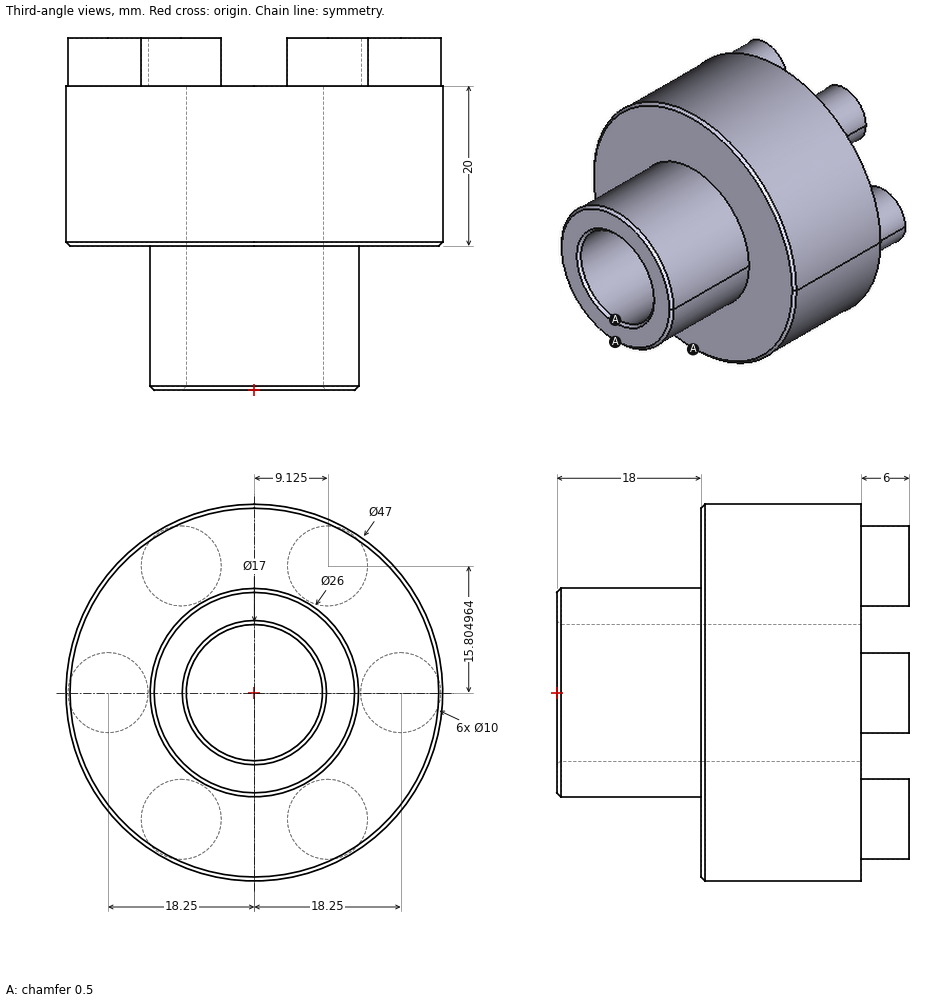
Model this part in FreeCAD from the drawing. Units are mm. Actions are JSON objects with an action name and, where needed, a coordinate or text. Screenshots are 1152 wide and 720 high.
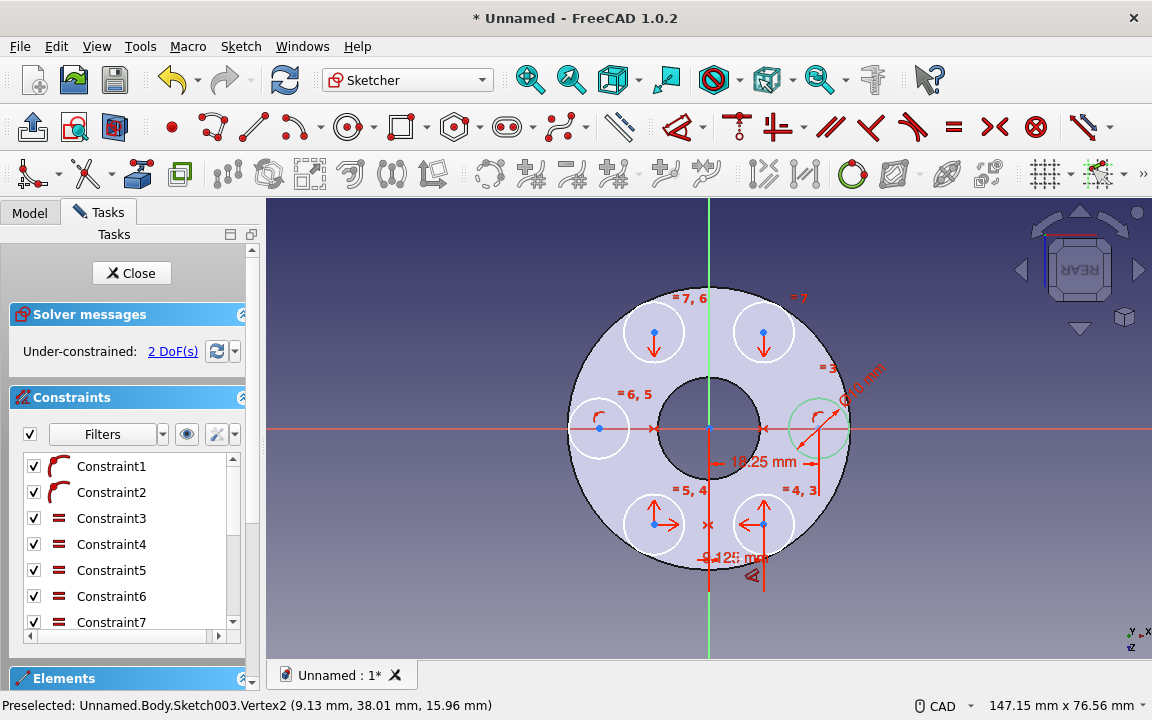
{"action": "left_click", "coordinate": [599, 429]}
{"action": "left_click", "coordinate": [654, 463]}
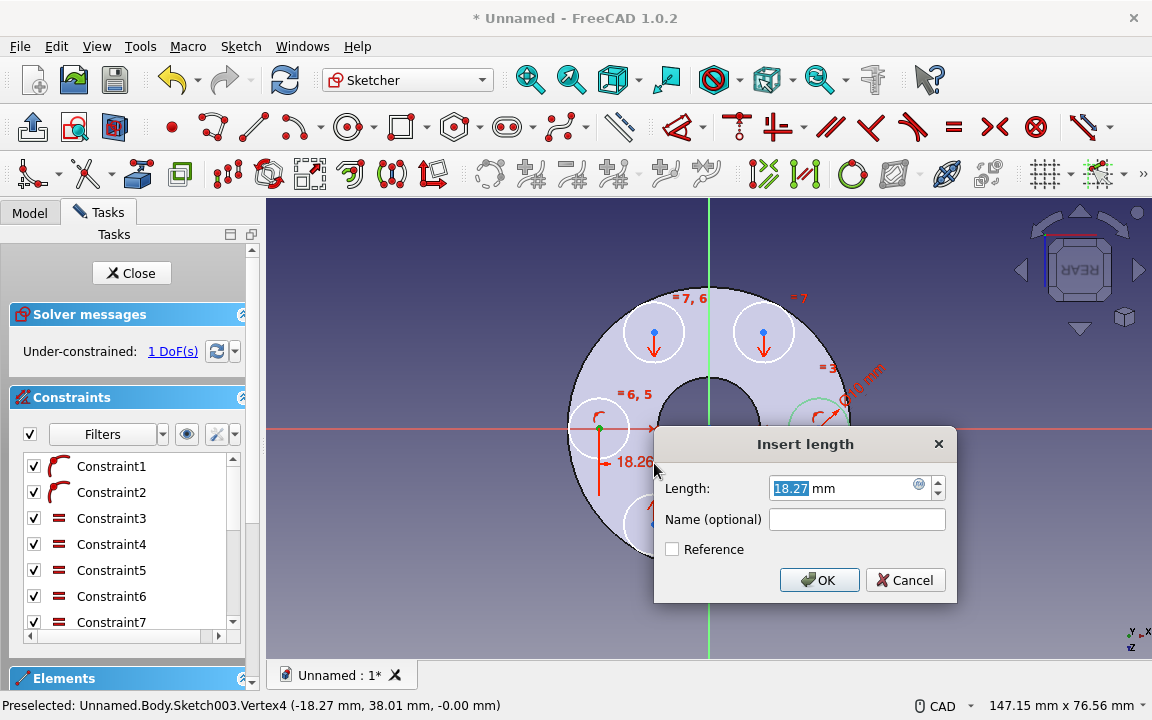
{"action": "type", "text": "18.25"}
{"action": "key", "text": "Return"}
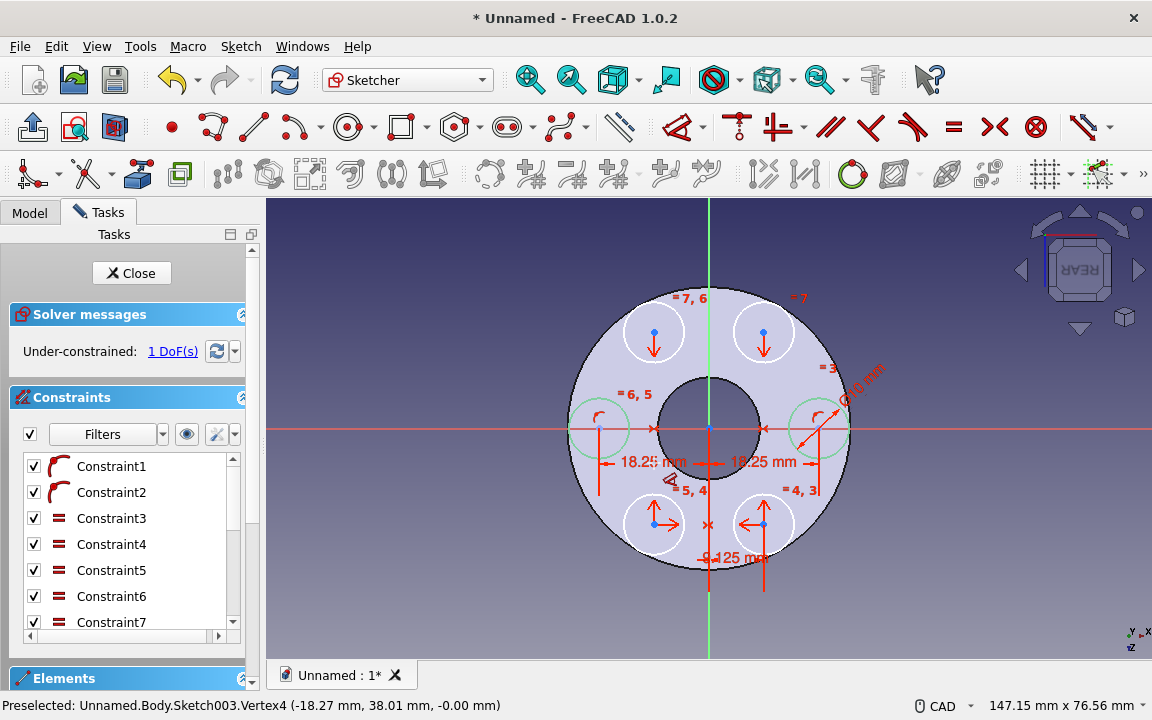
{"action": "left_click", "coordinate": [764, 525]}
{"action": "left_click", "coordinate": [822, 499]}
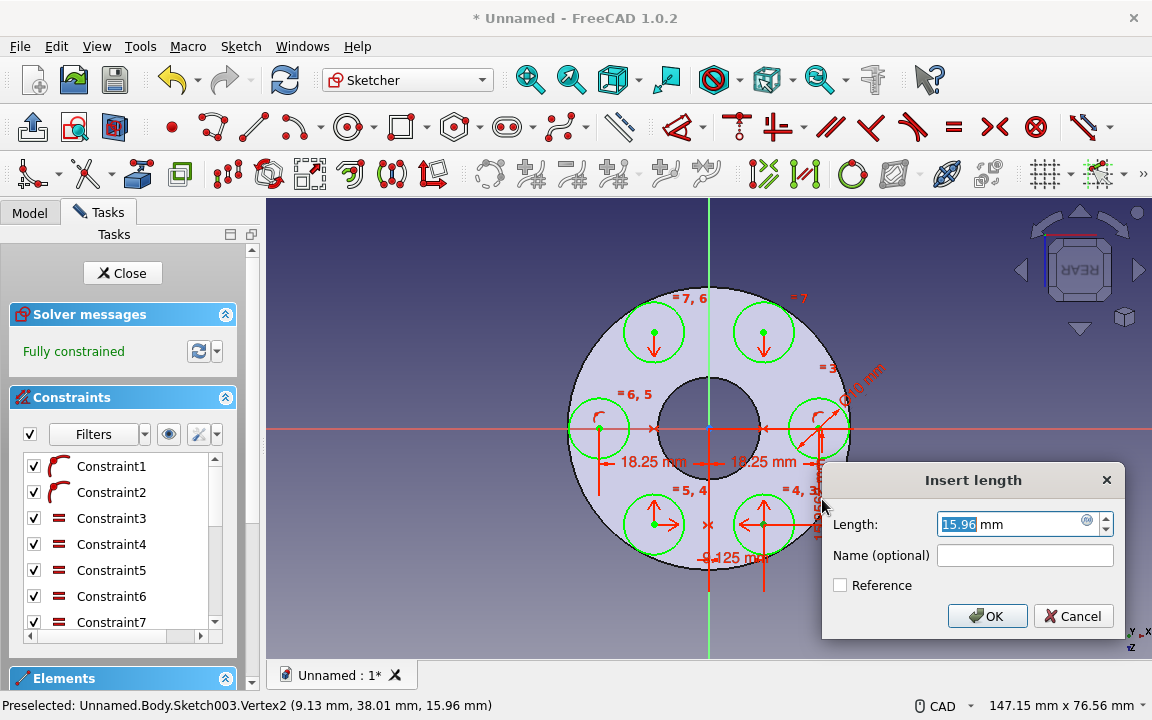
{"action": "type", "text": "15.804964"}
{"action": "key", "text": "Return"}
{"action": "key", "text": "Escape"}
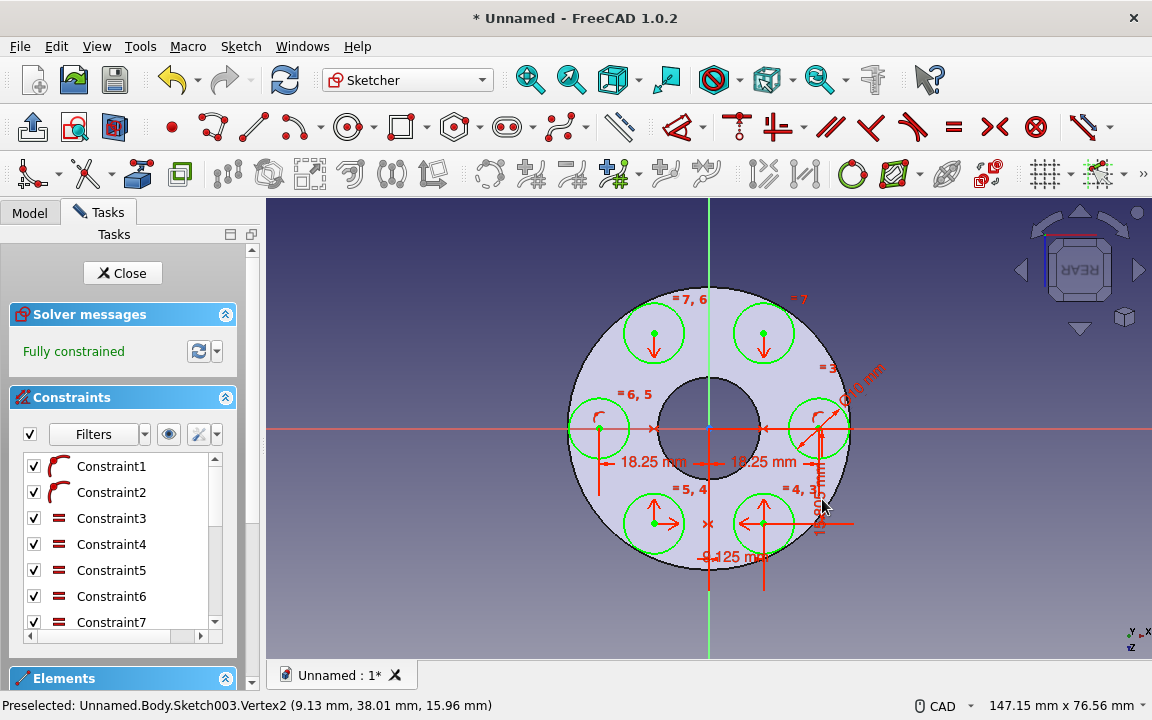
{"action": "left_click", "coordinate": [123, 273]}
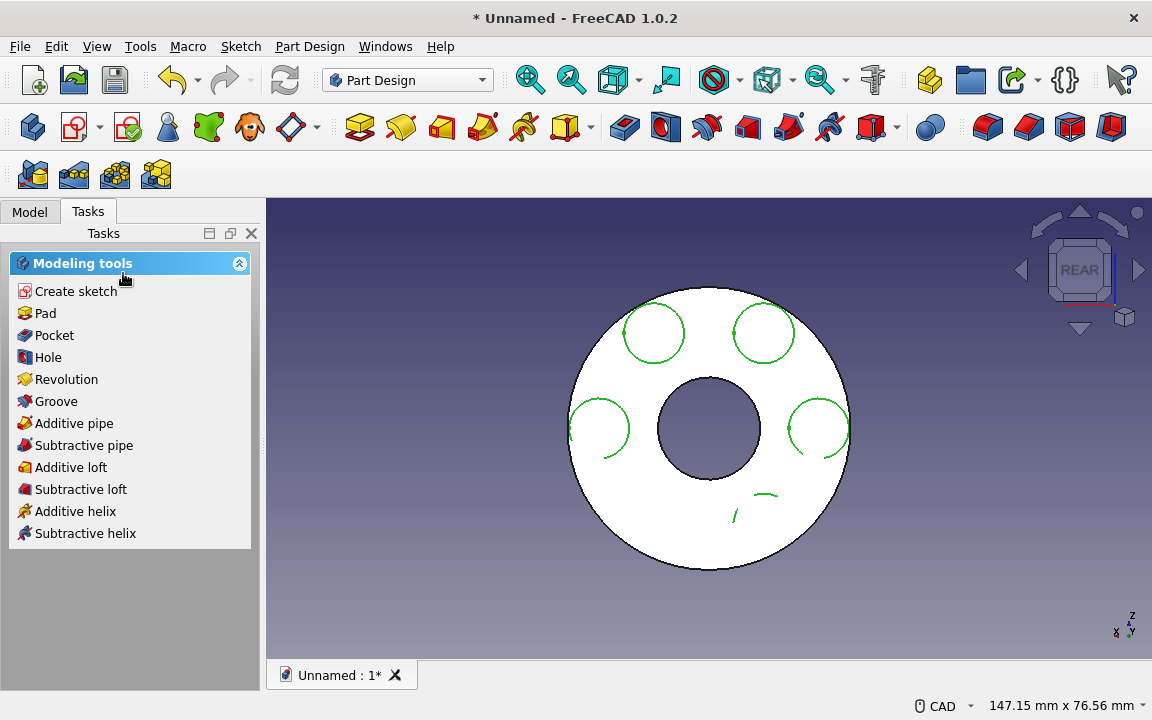
{"action": "left_click", "coordinate": [360, 128]}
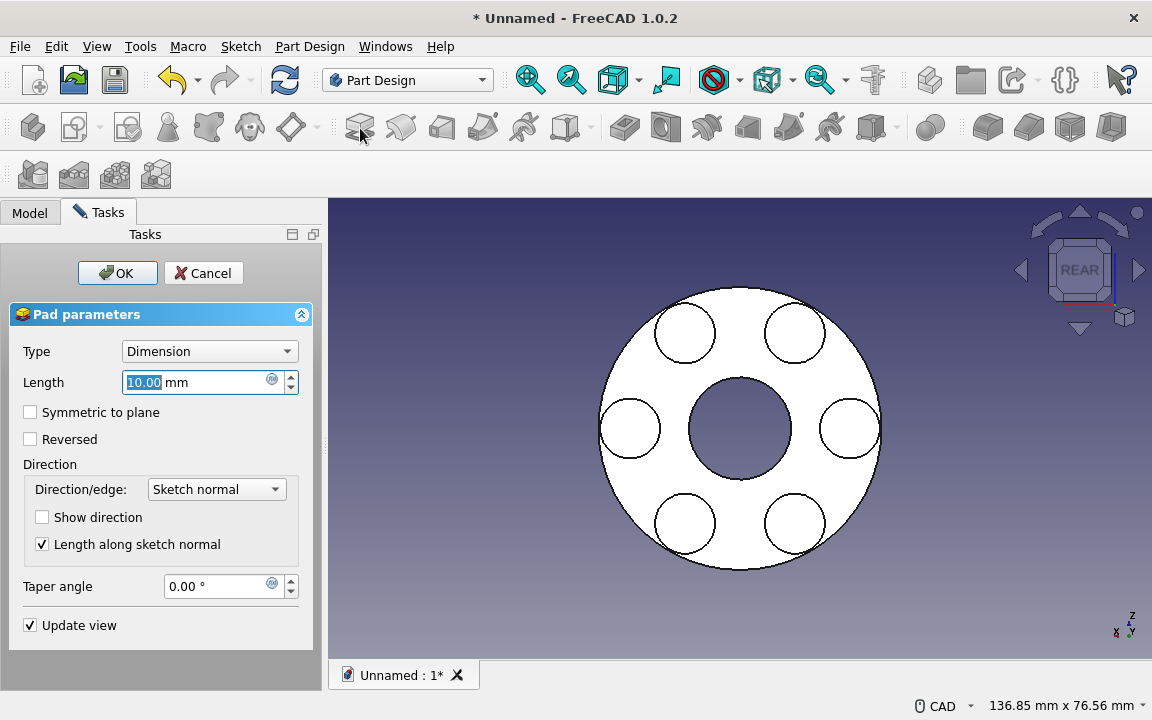
{"action": "type", "text": "6"}
{"action": "key", "text": "Tab"}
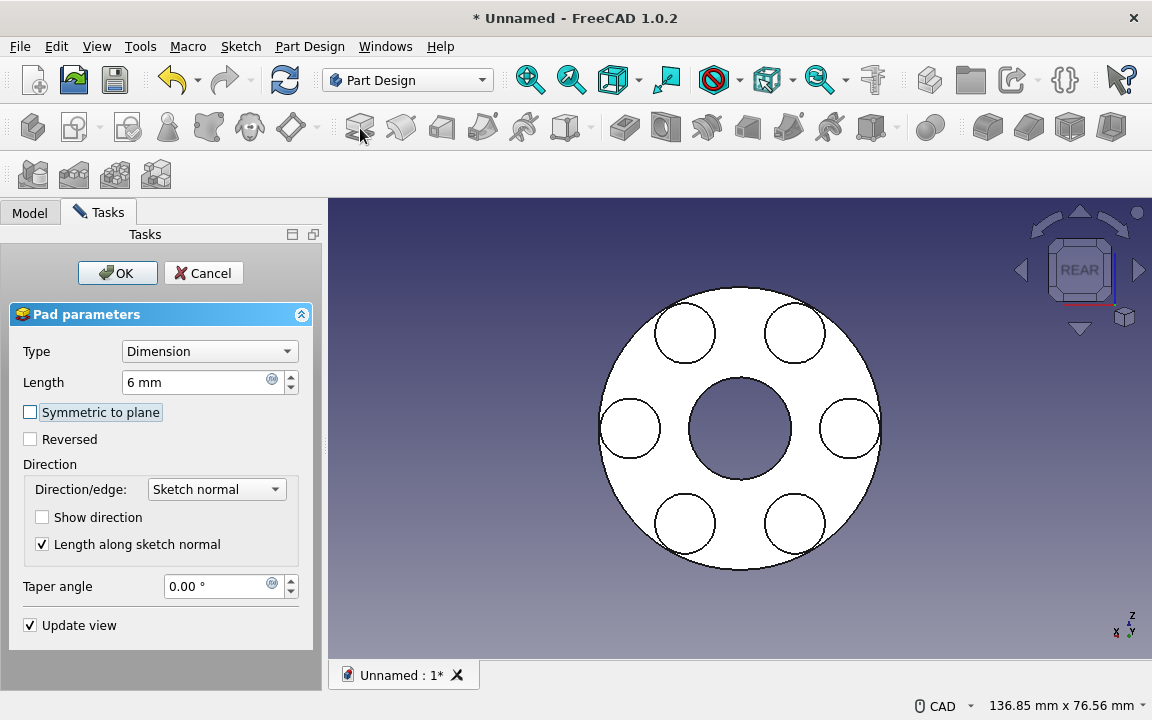
{"action": "left_click", "coordinate": [118, 273]}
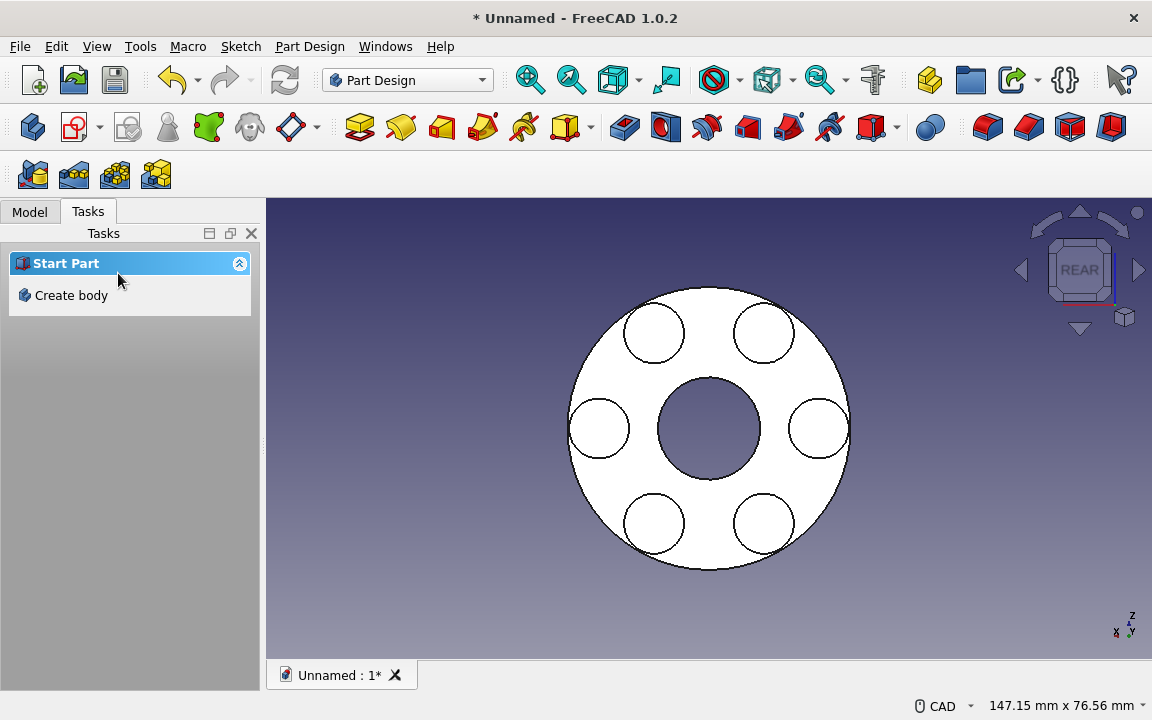
{"action": "key", "text": "0"}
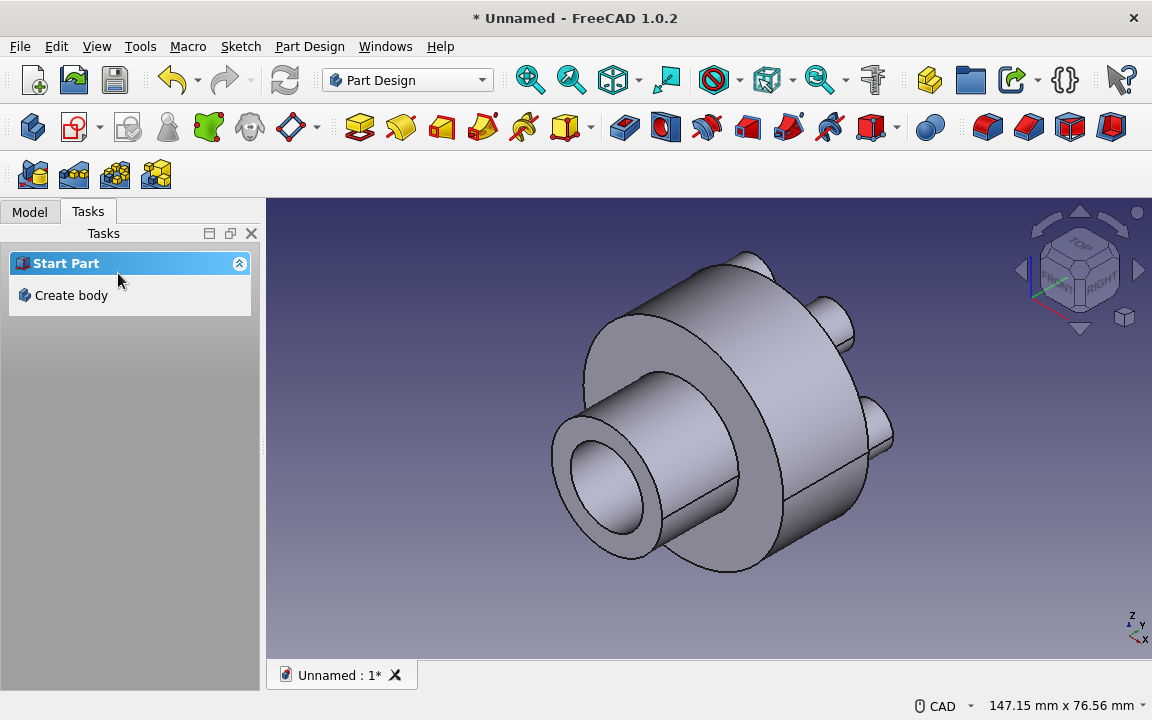
{"action": "left_click", "coordinate": [531, 80]}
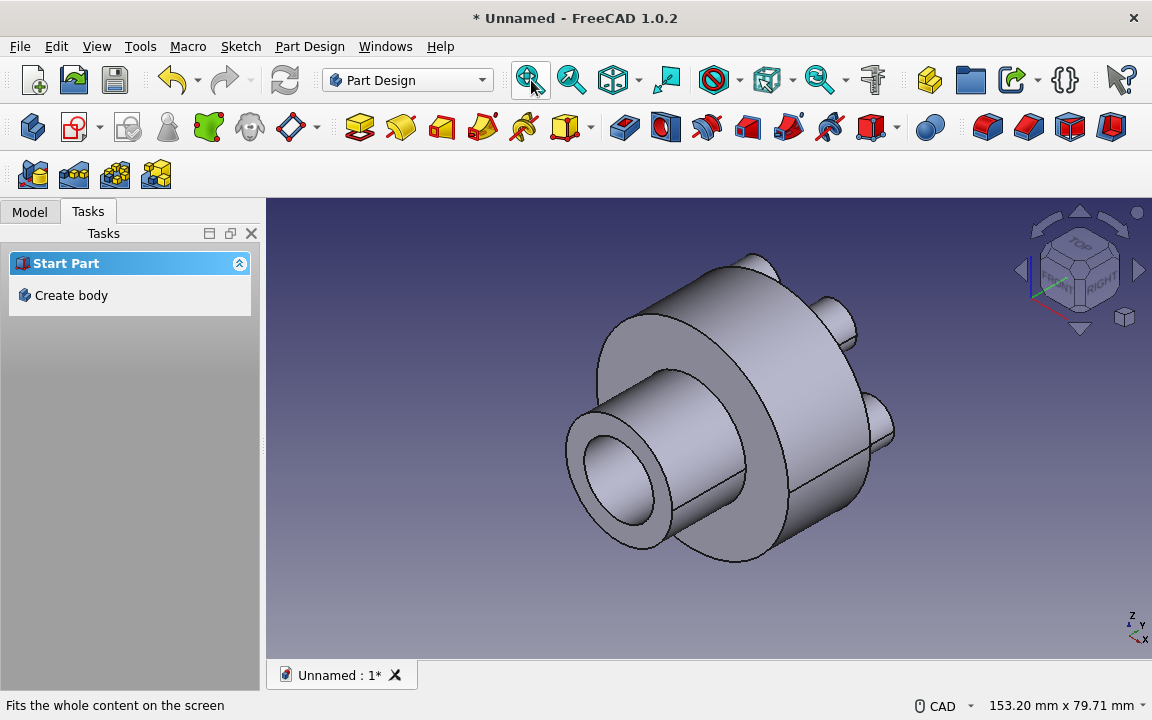
{"action": "left_click", "coordinate": [603, 412]}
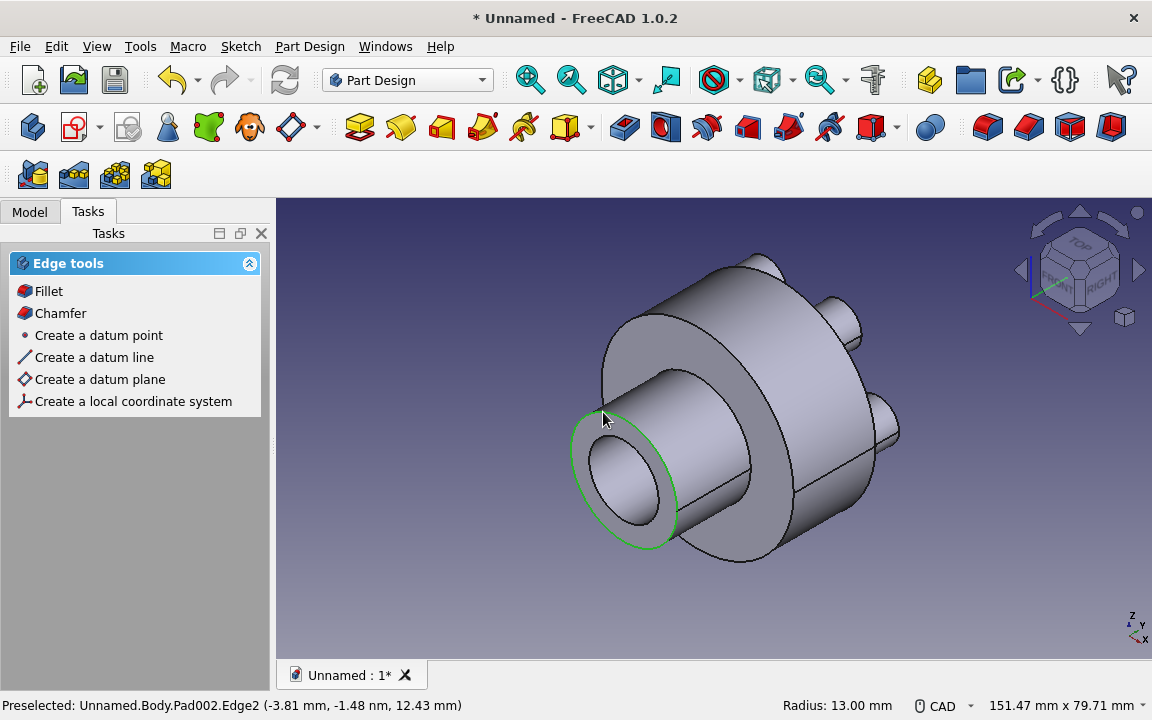
{"action": "left_click", "coordinate": [589, 459], "text": "ctrl"}